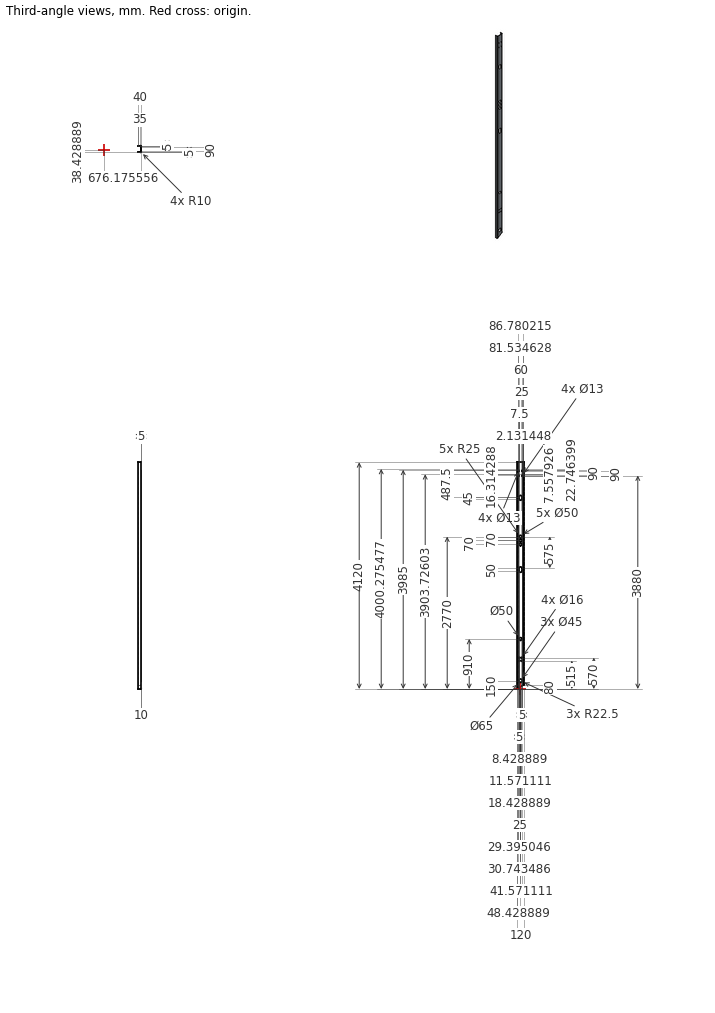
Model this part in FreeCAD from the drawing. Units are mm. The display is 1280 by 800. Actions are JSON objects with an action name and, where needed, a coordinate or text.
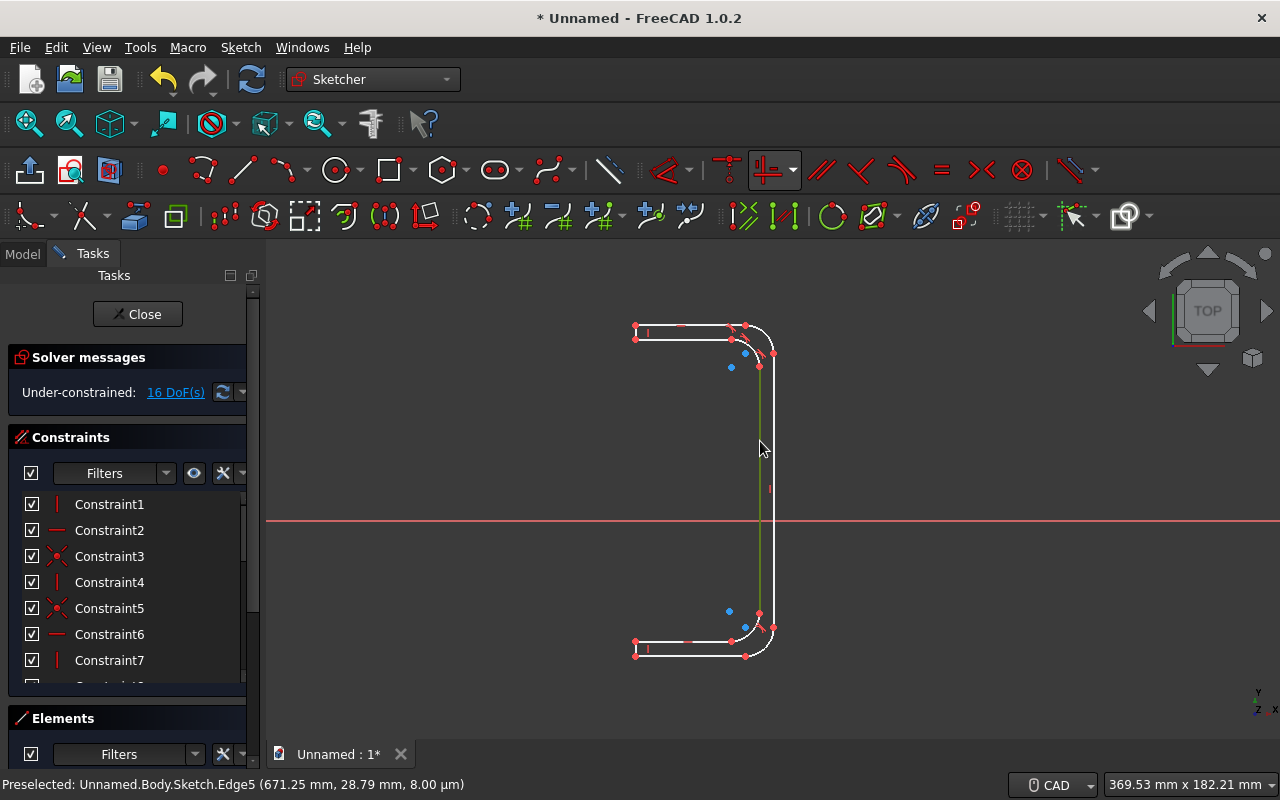
{"action": "left_click", "coordinate": [744, 343]}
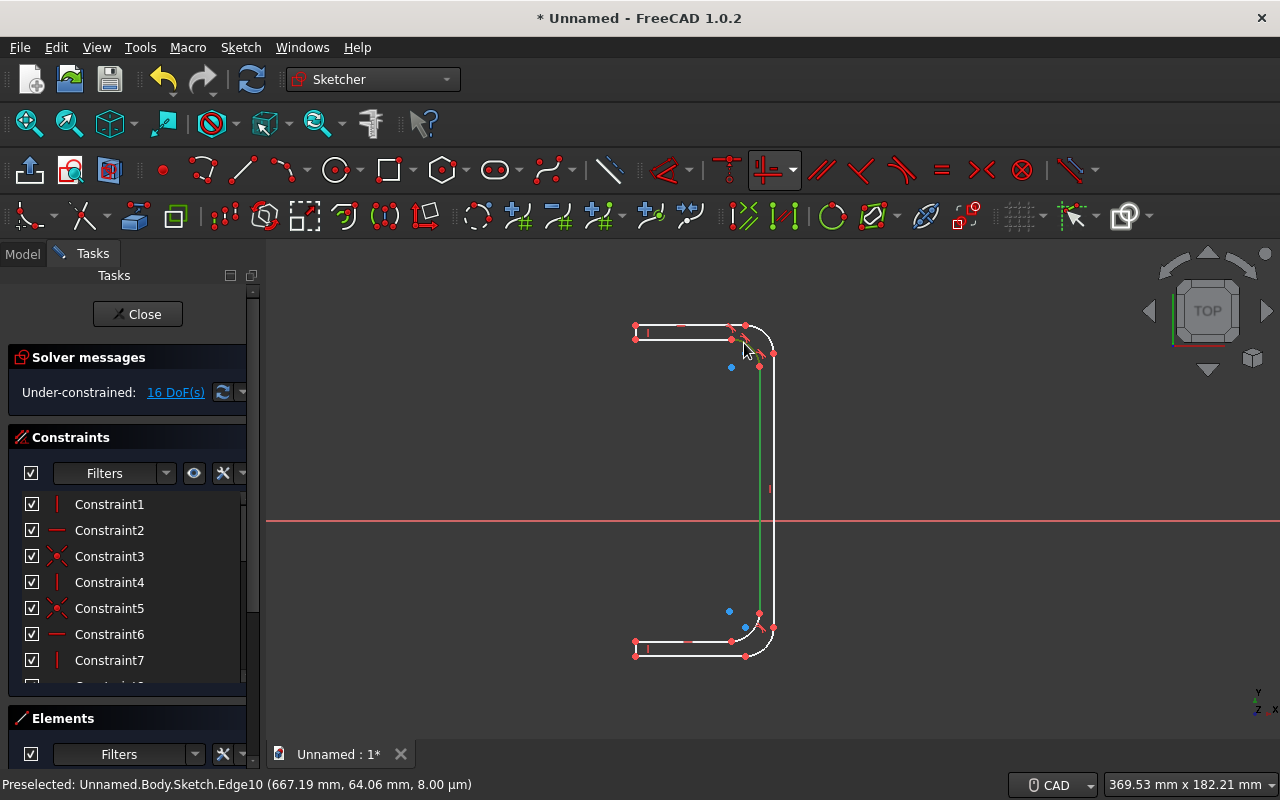
{"action": "left_click", "coordinate": [902, 170]}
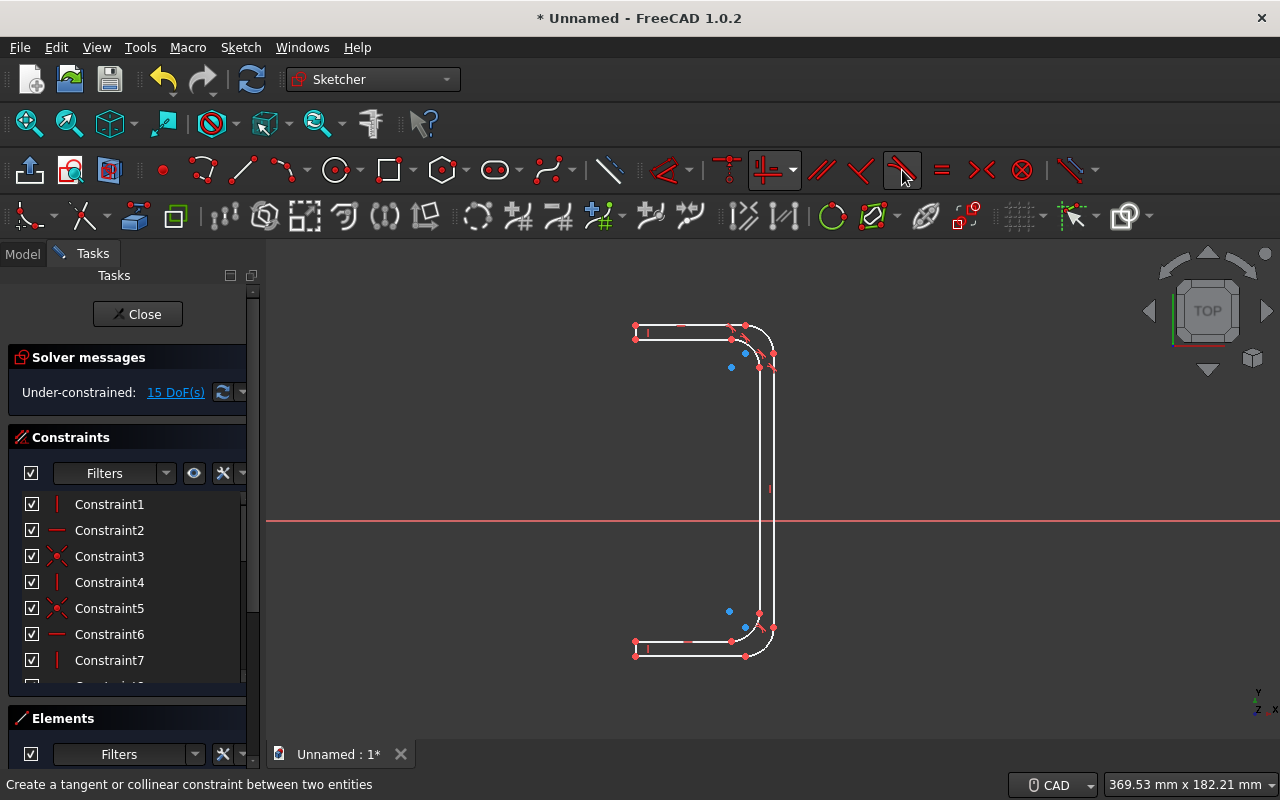
{"action": "left_click", "coordinate": [760, 441]}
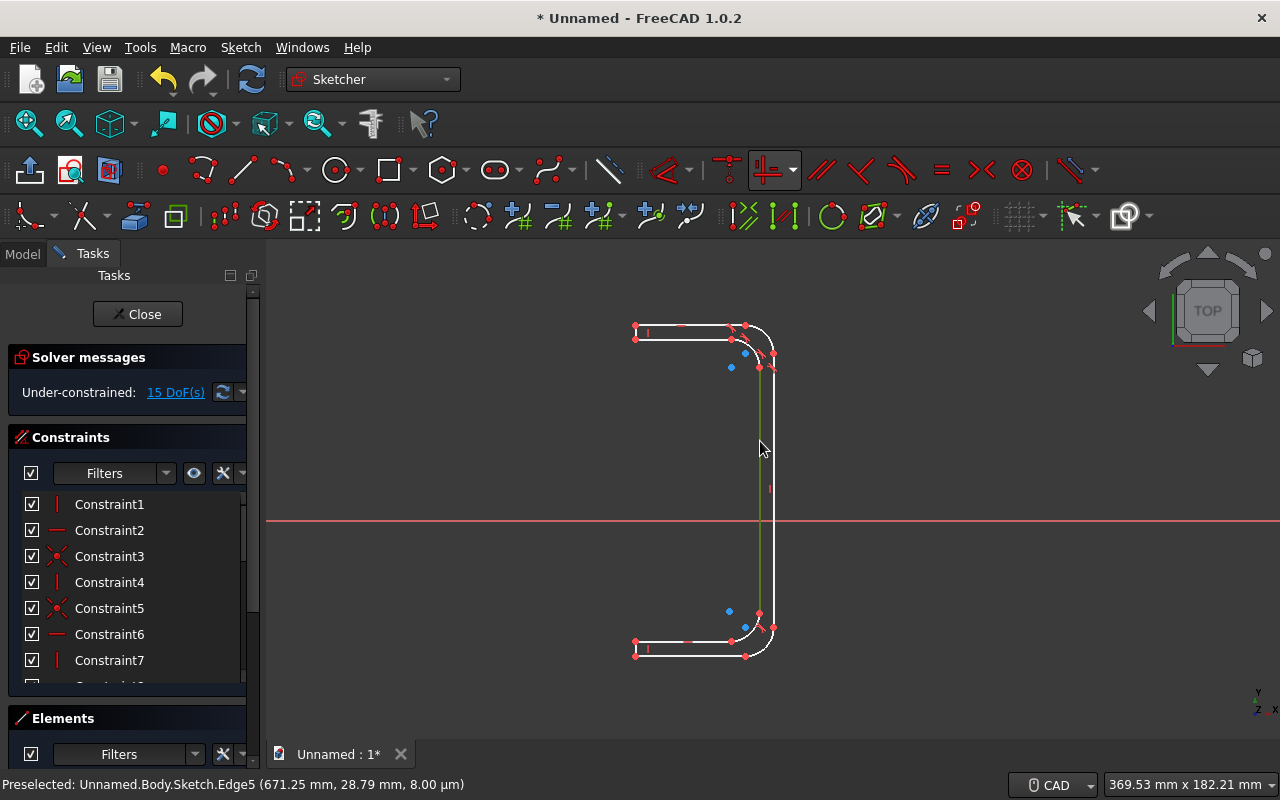
{"action": "left_click", "coordinate": [744, 638]}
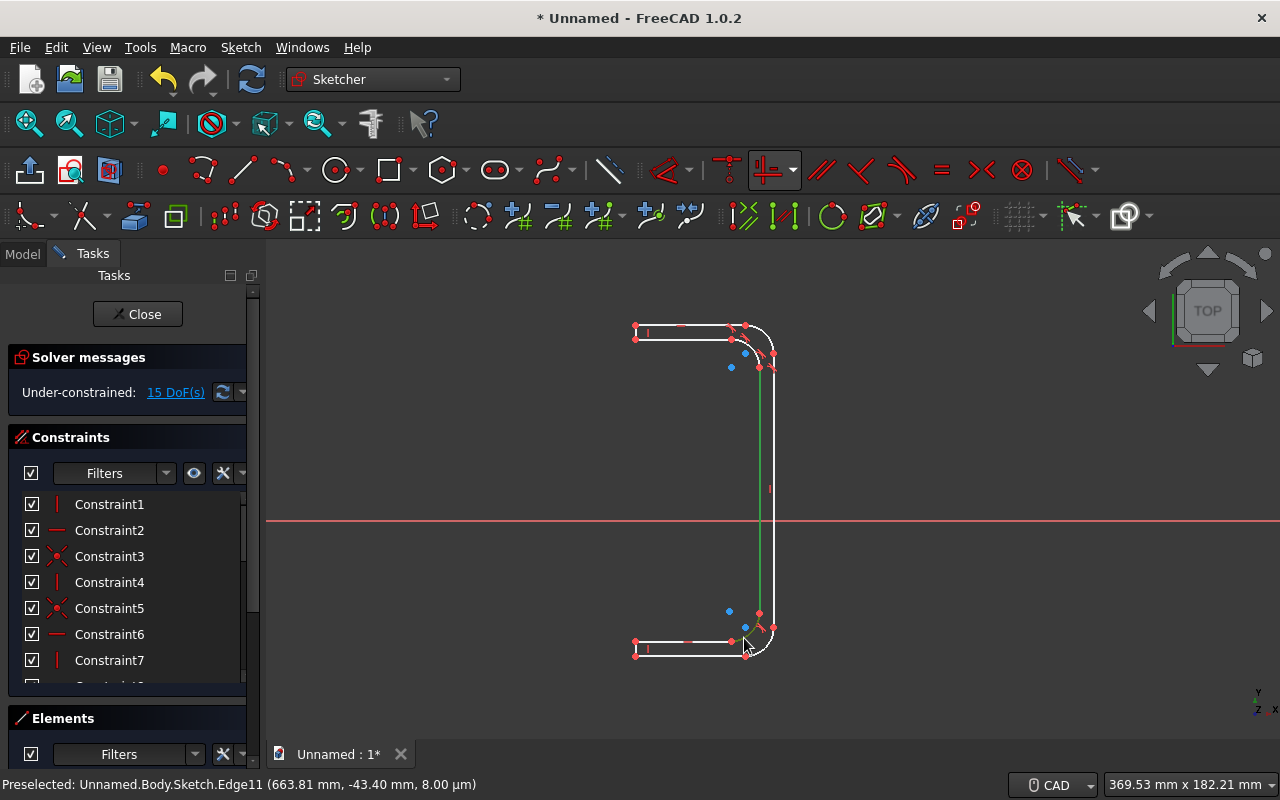
{"action": "key", "text": "t"}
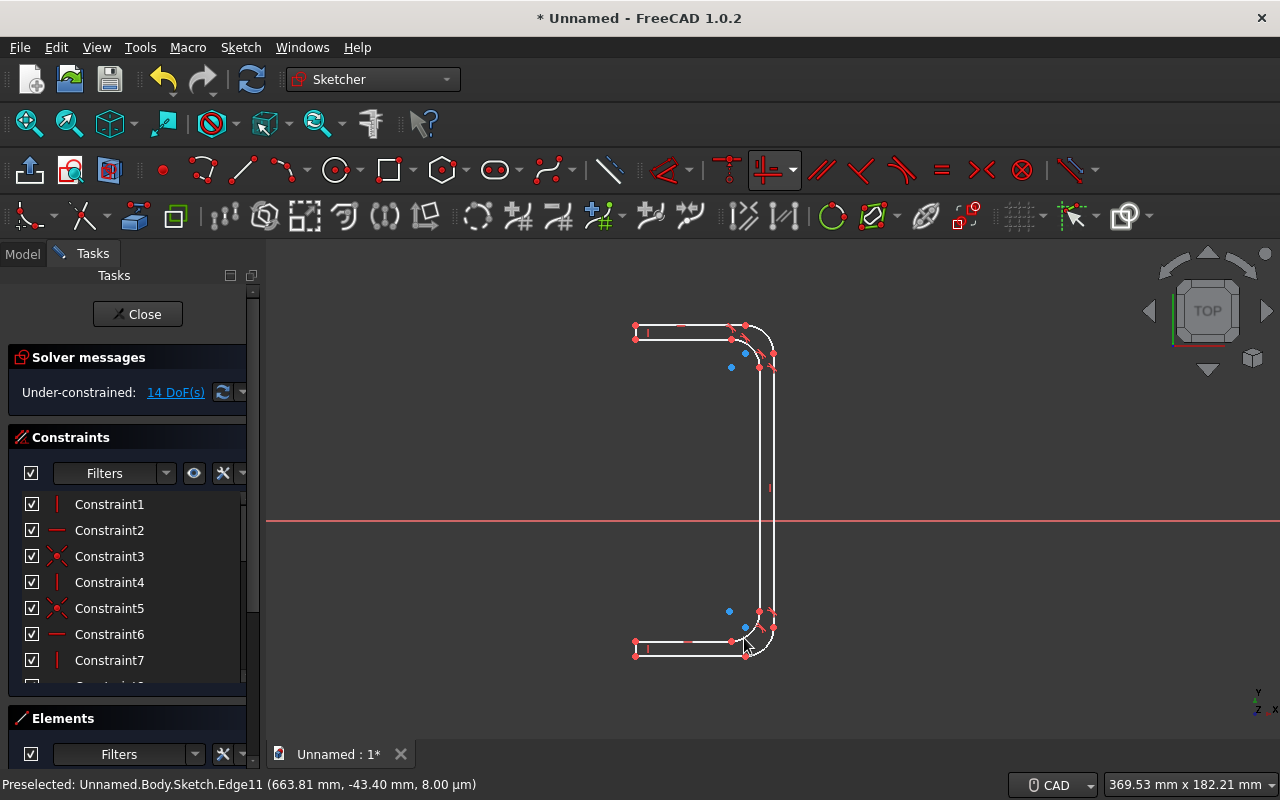
{"action": "left_click", "coordinate": [703, 642]}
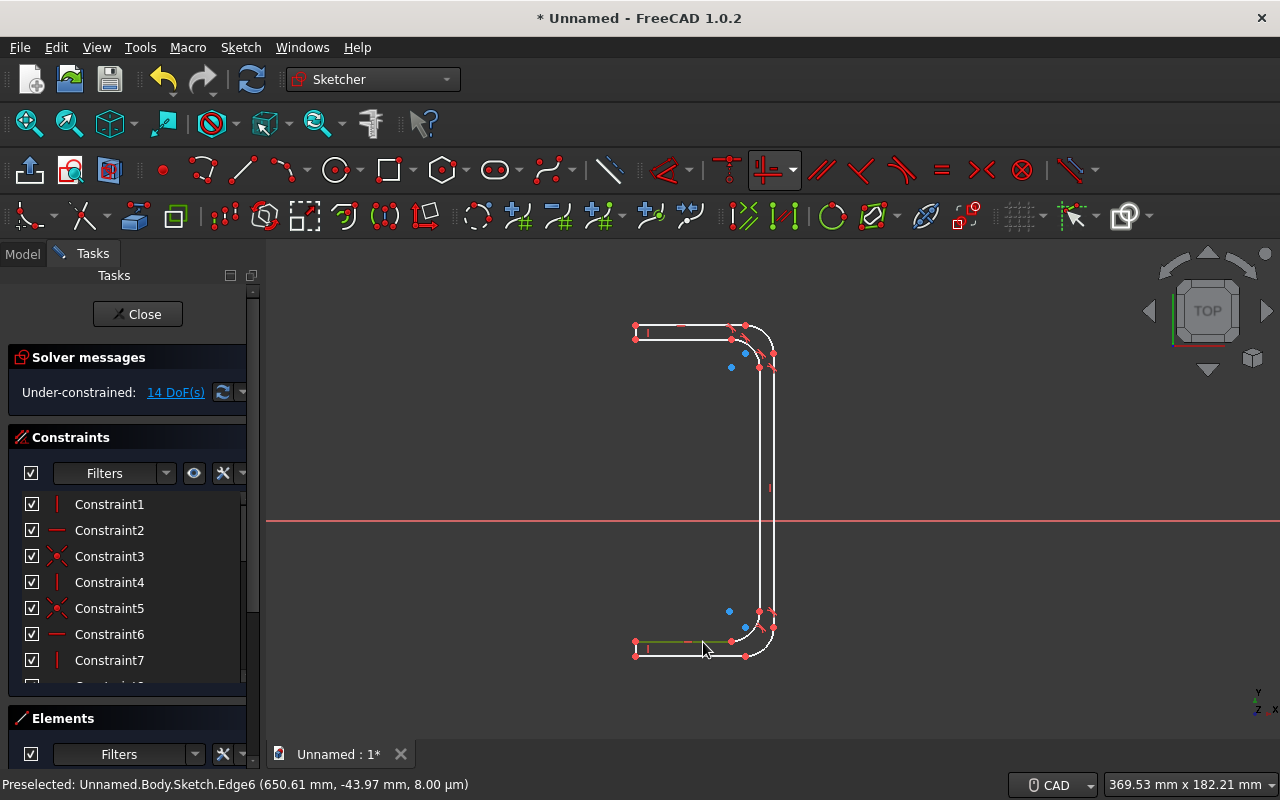
{"action": "left_click", "coordinate": [745, 638]}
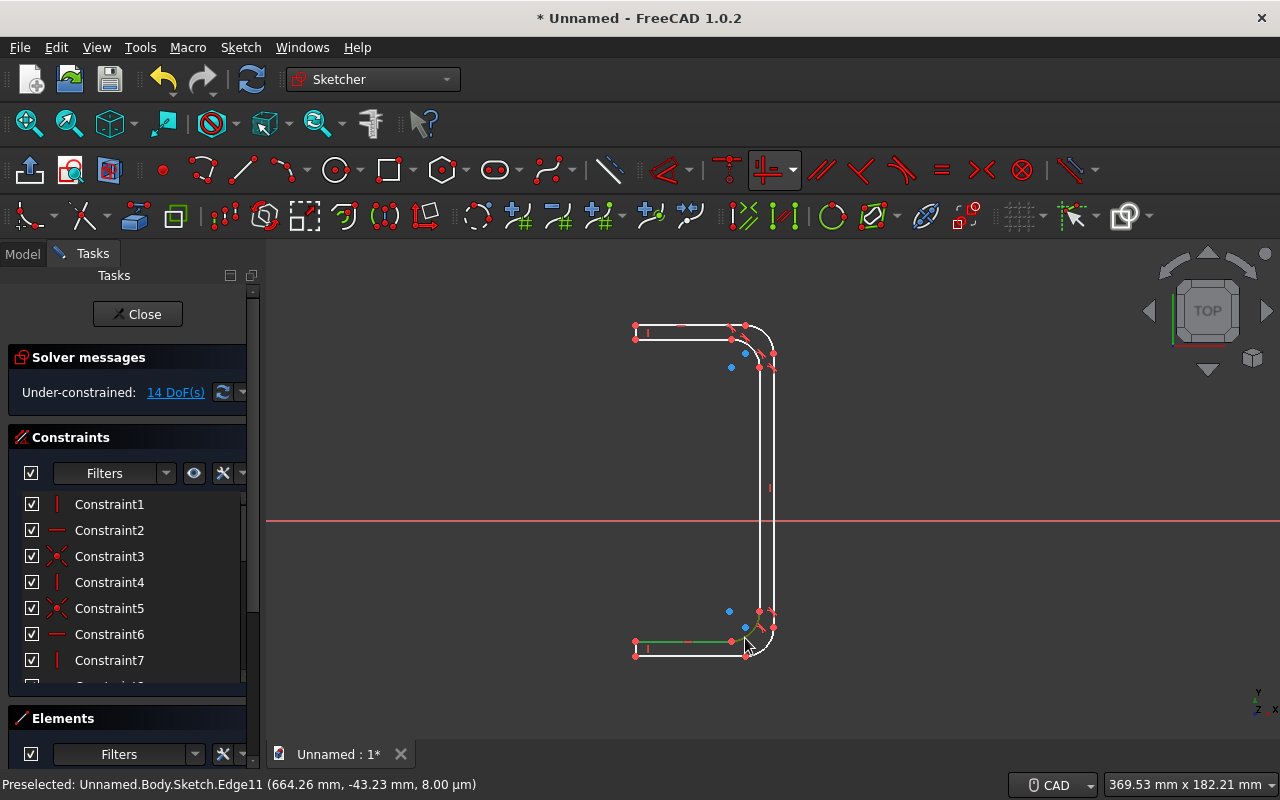
{"action": "key", "text": "t"}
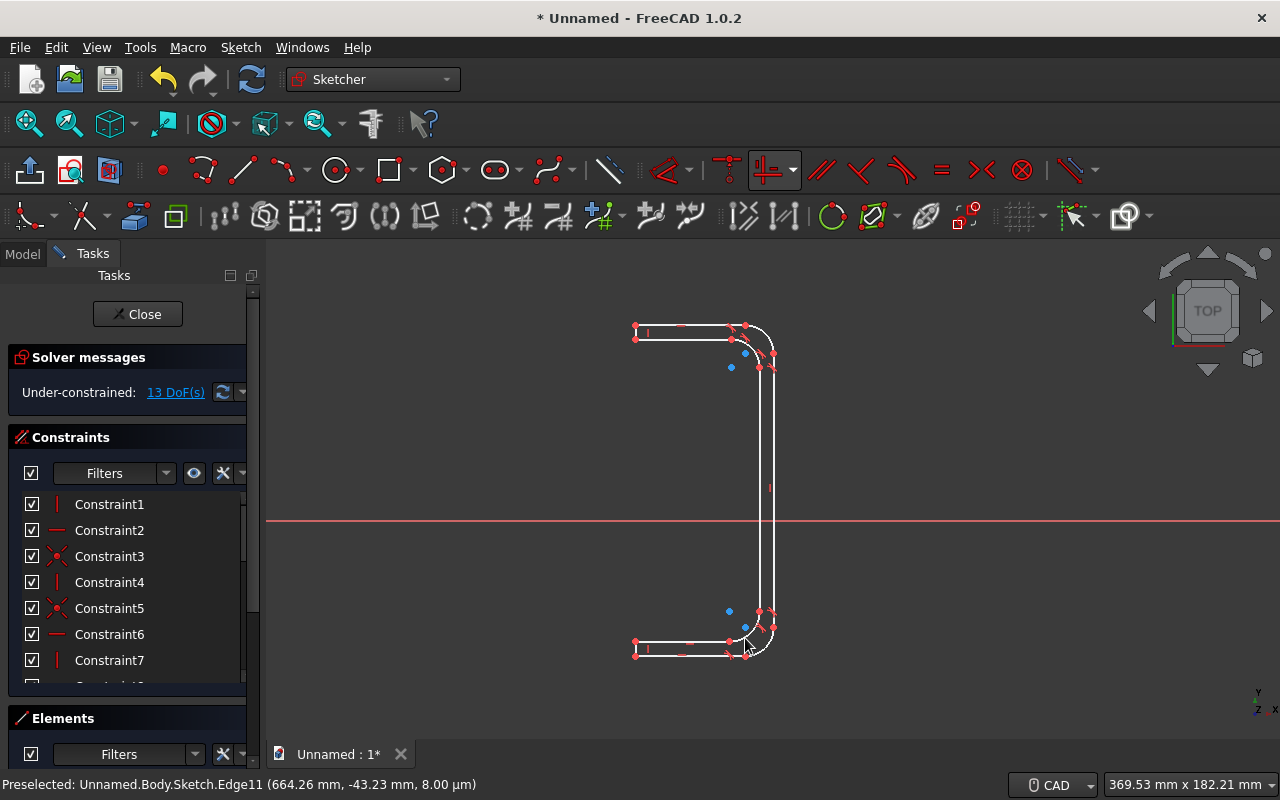
{"action": "left_click", "coordinate": [669, 656]}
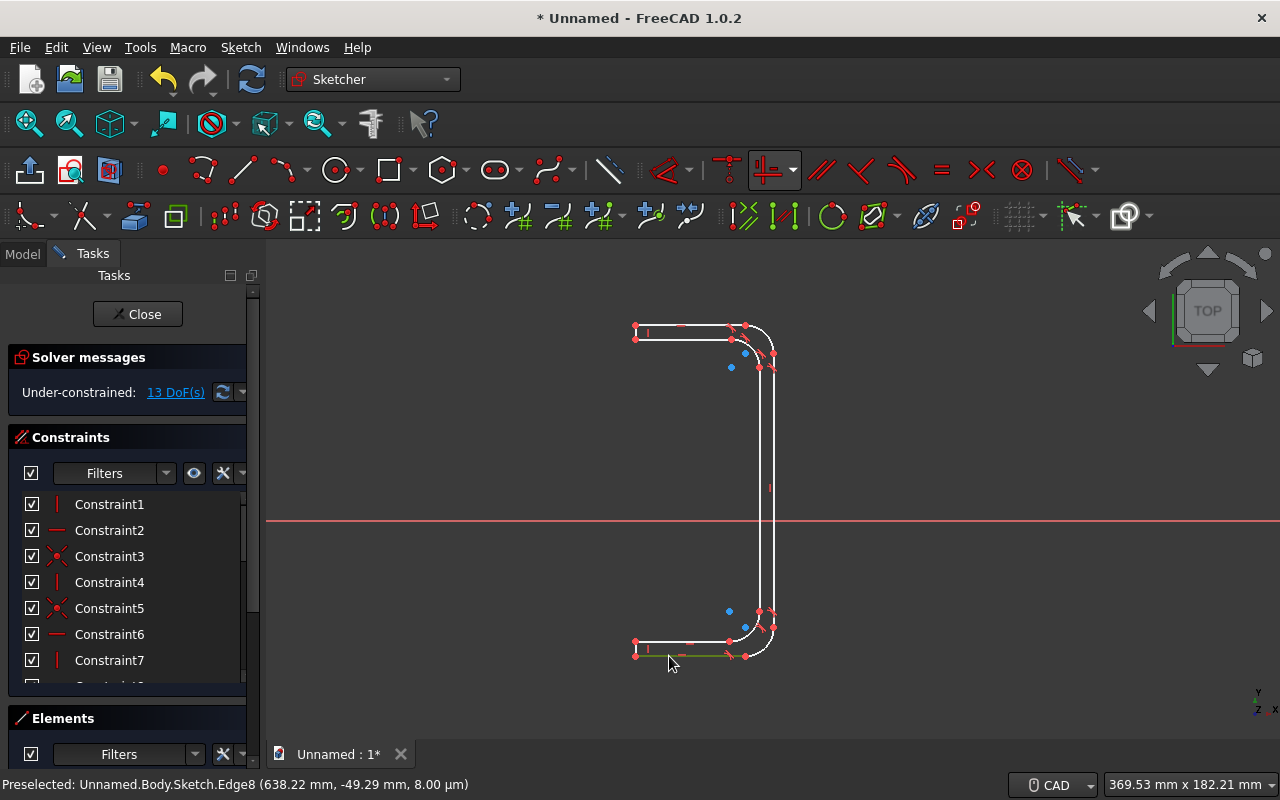
{"action": "left_click", "coordinate": [758, 653]}